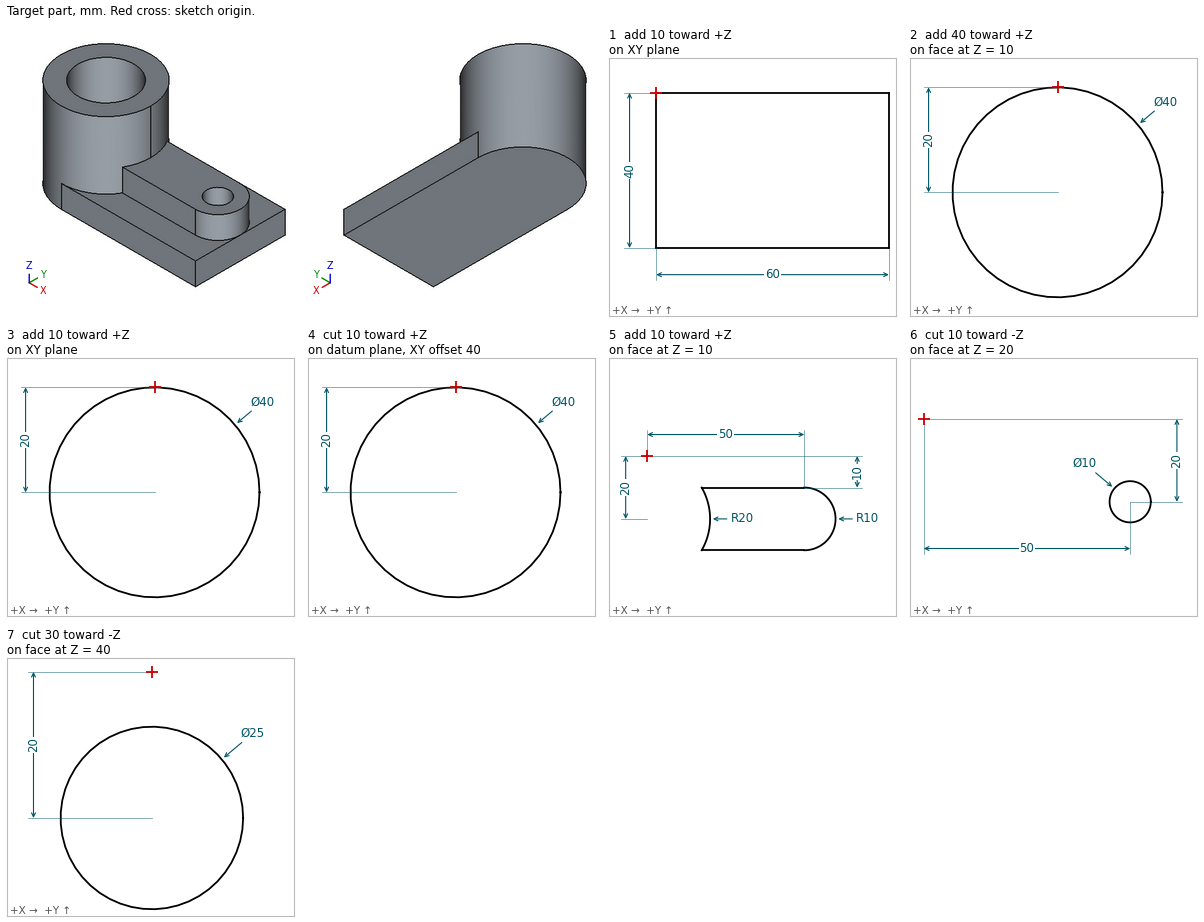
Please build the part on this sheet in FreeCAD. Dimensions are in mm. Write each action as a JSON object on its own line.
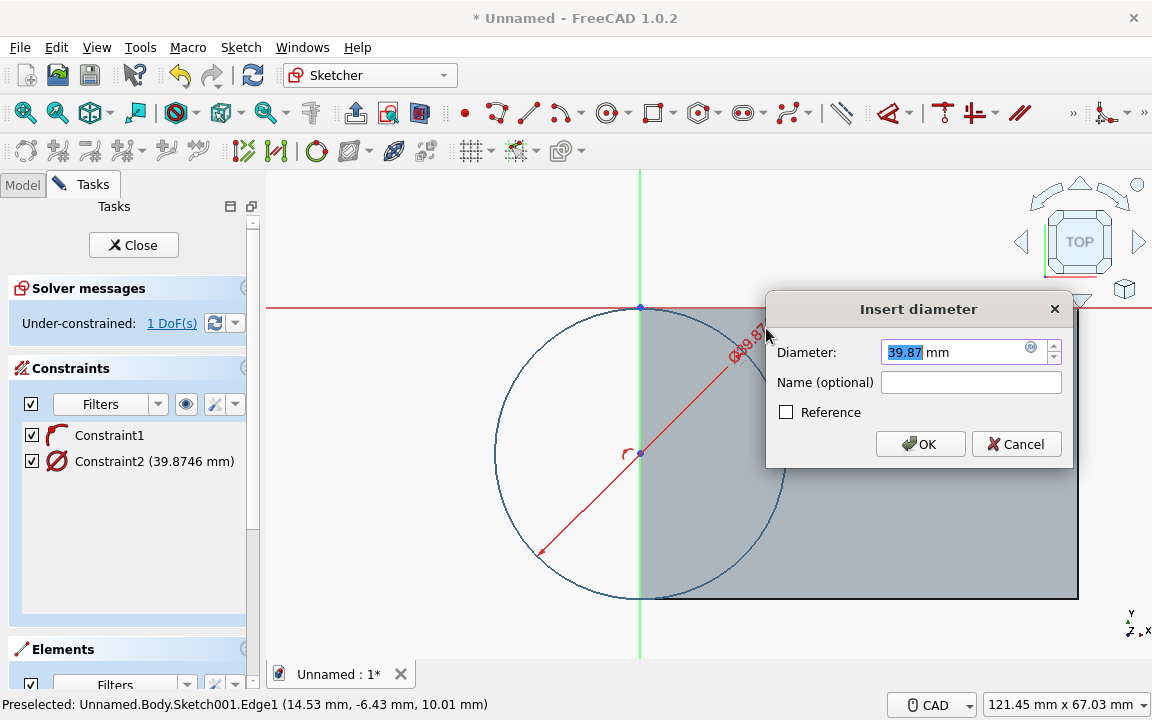
{"action": "type", "text": "40"}
{"action": "key", "text": "Return"}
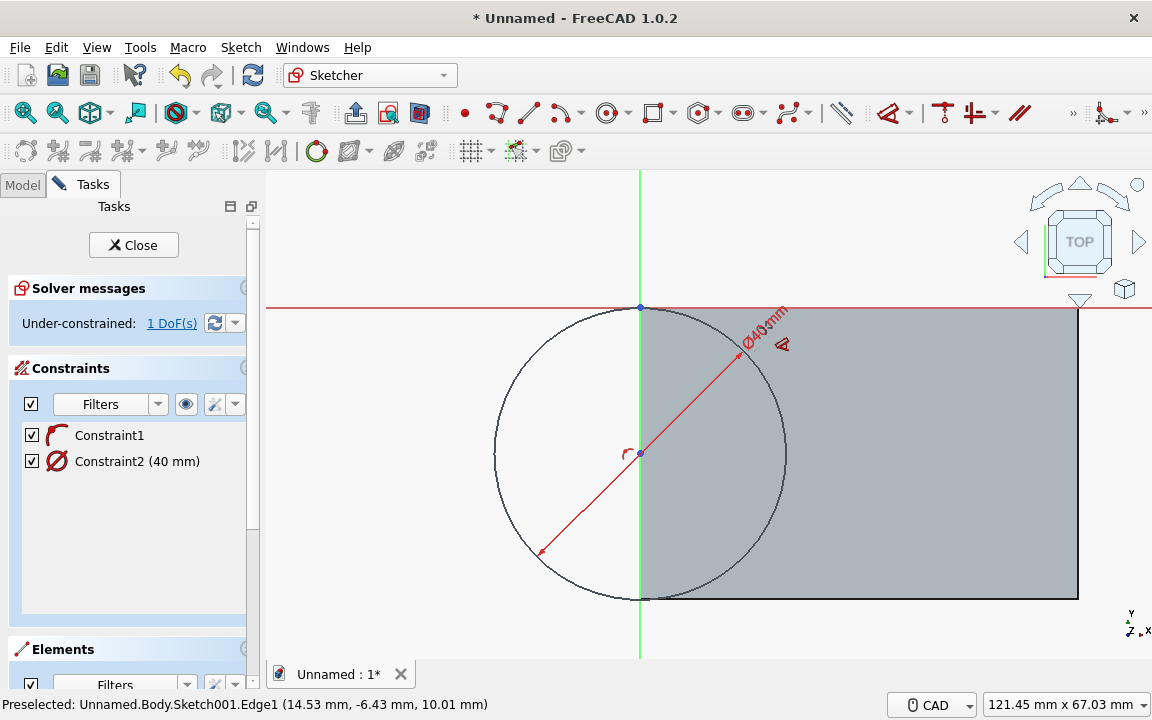
{"action": "left_click", "coordinate": [640, 454]}
{"action": "left_click", "coordinate": [674, 381]}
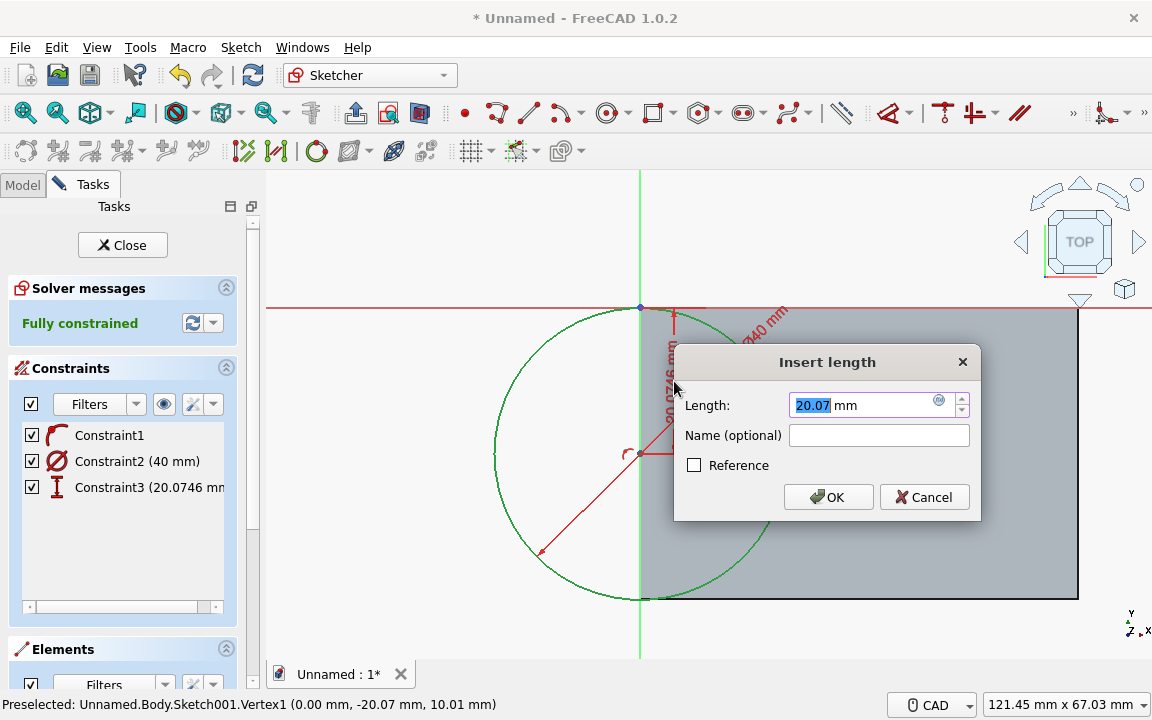
{"action": "type", "text": "20"}
{"action": "key", "text": "Return"}
{"action": "key", "text": "Escape"}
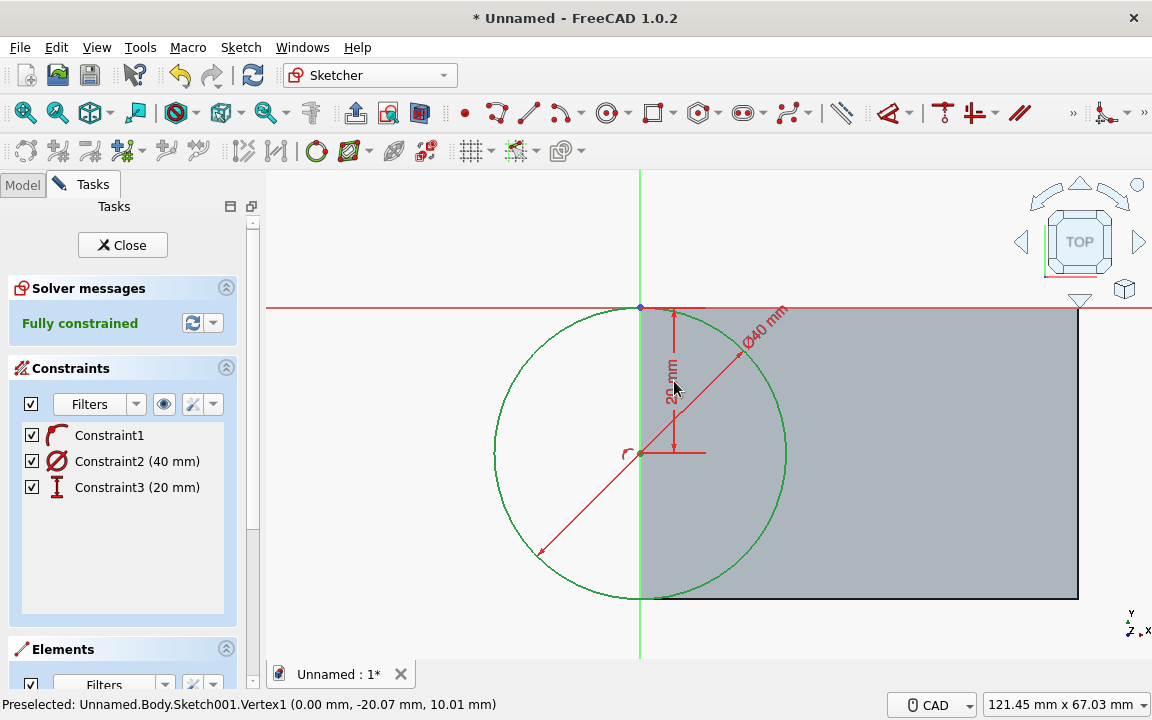
{"action": "left_click", "coordinate": [123, 245]}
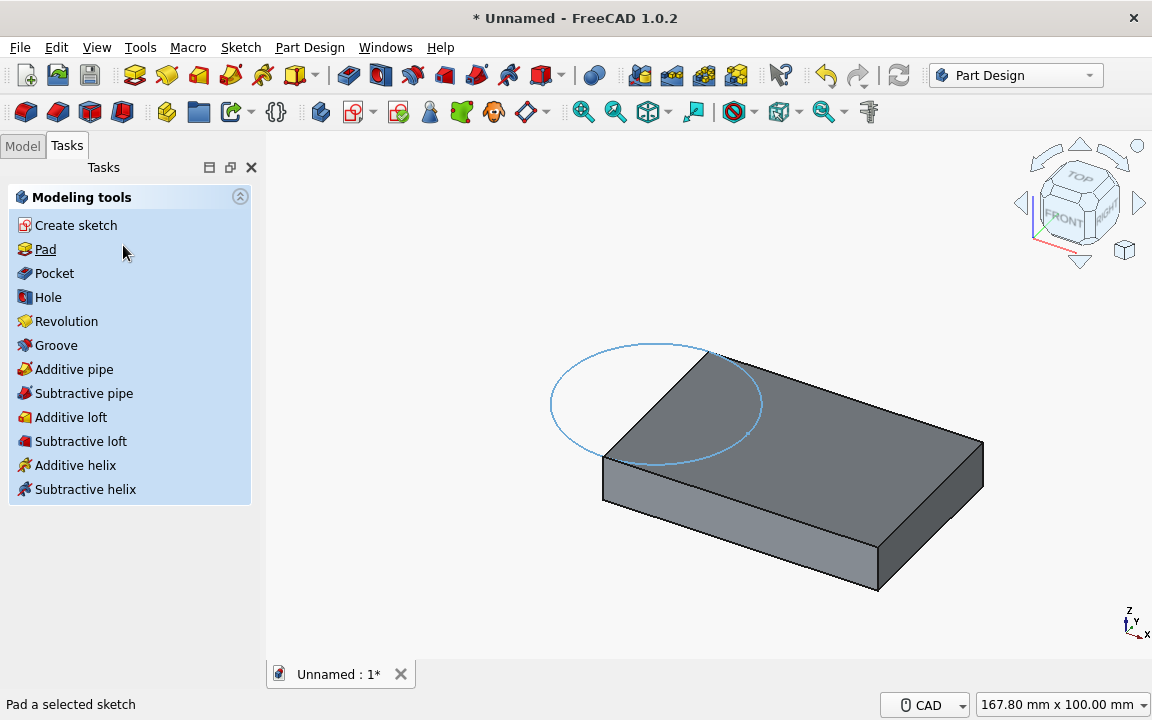
{"action": "left_click", "coordinate": [136, 76]}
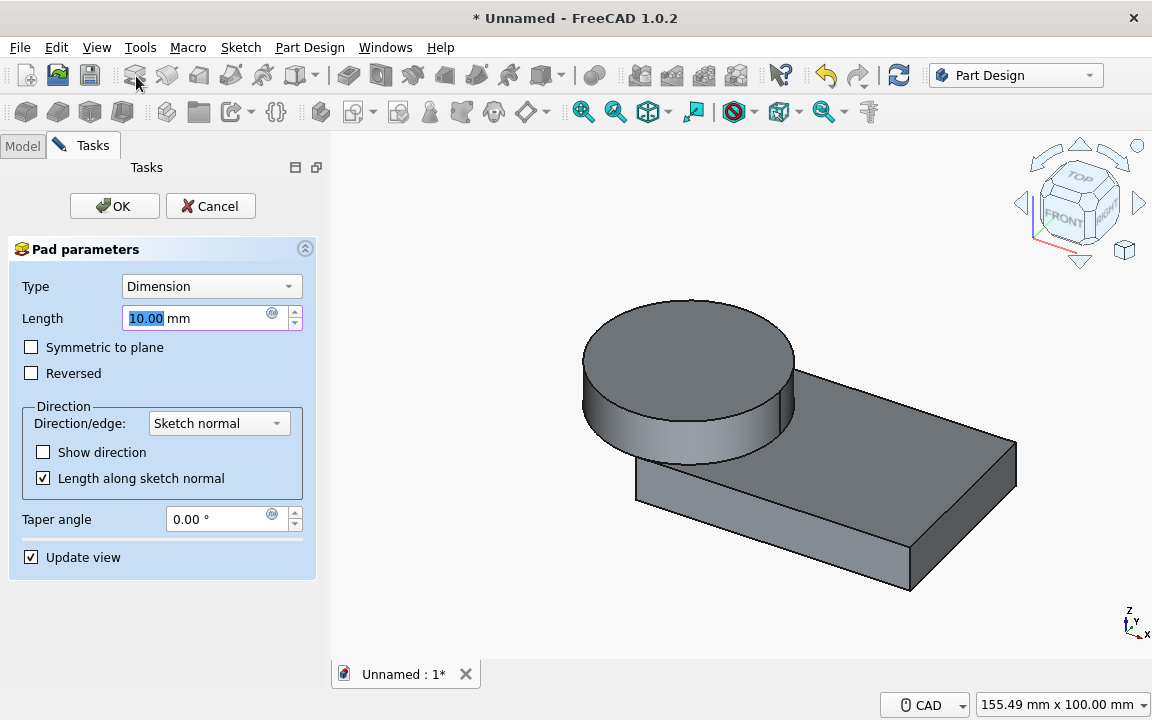
{"action": "type", "text": "40"}
{"action": "key", "text": "Tab"}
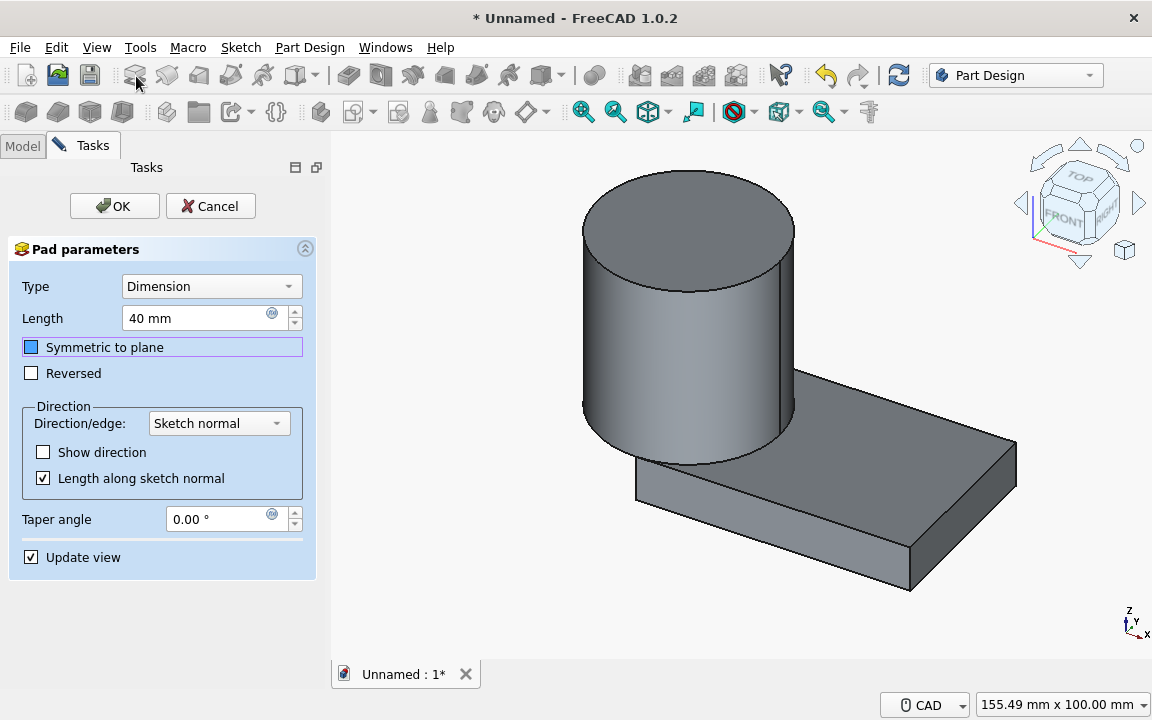
{"action": "left_click", "coordinate": [115, 206]}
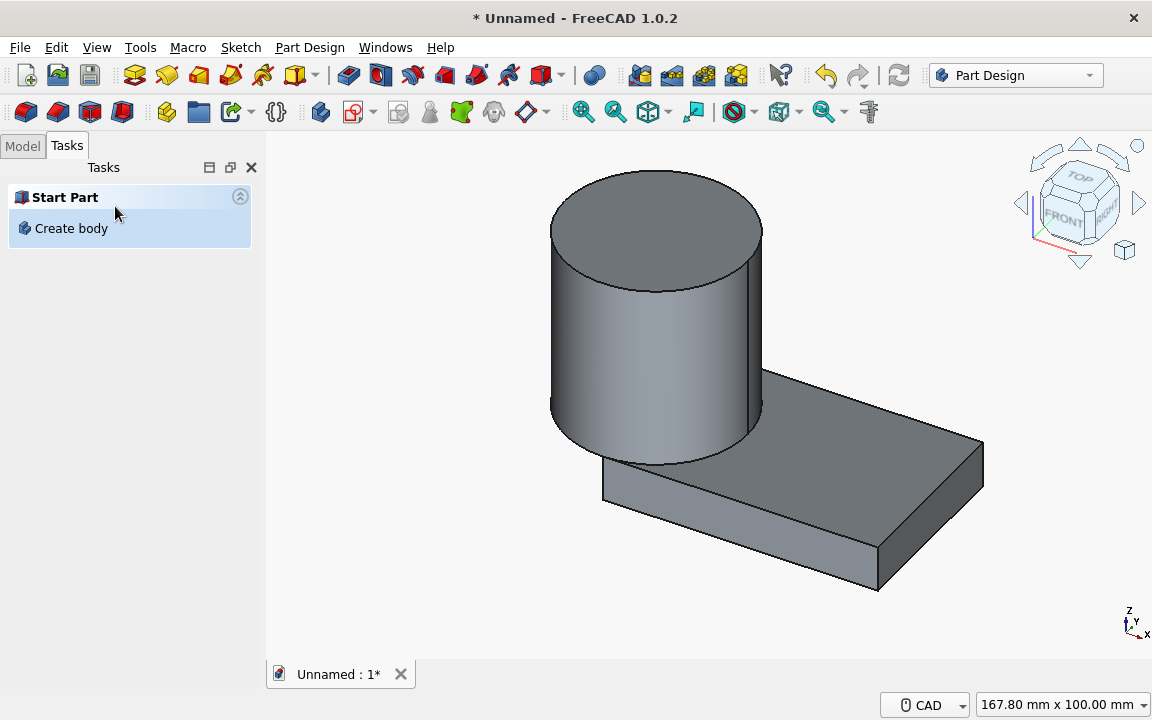
{"action": "left_click", "coordinate": [354, 112]}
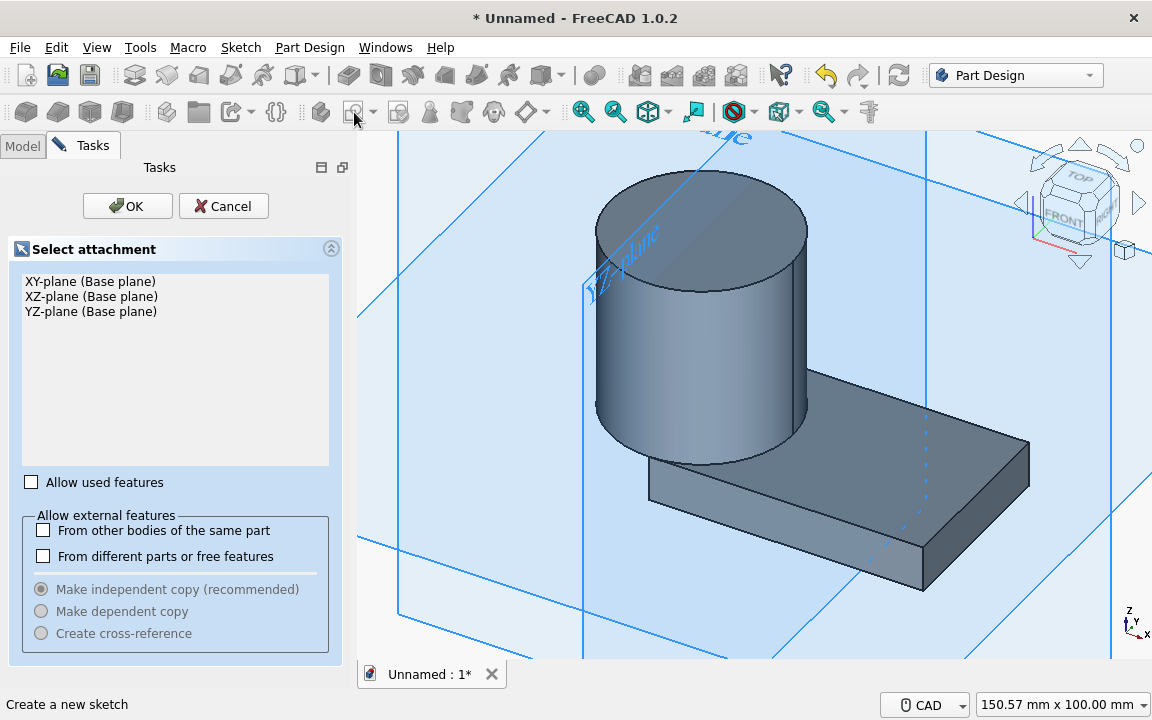
{"action": "left_click", "coordinate": [82, 282]}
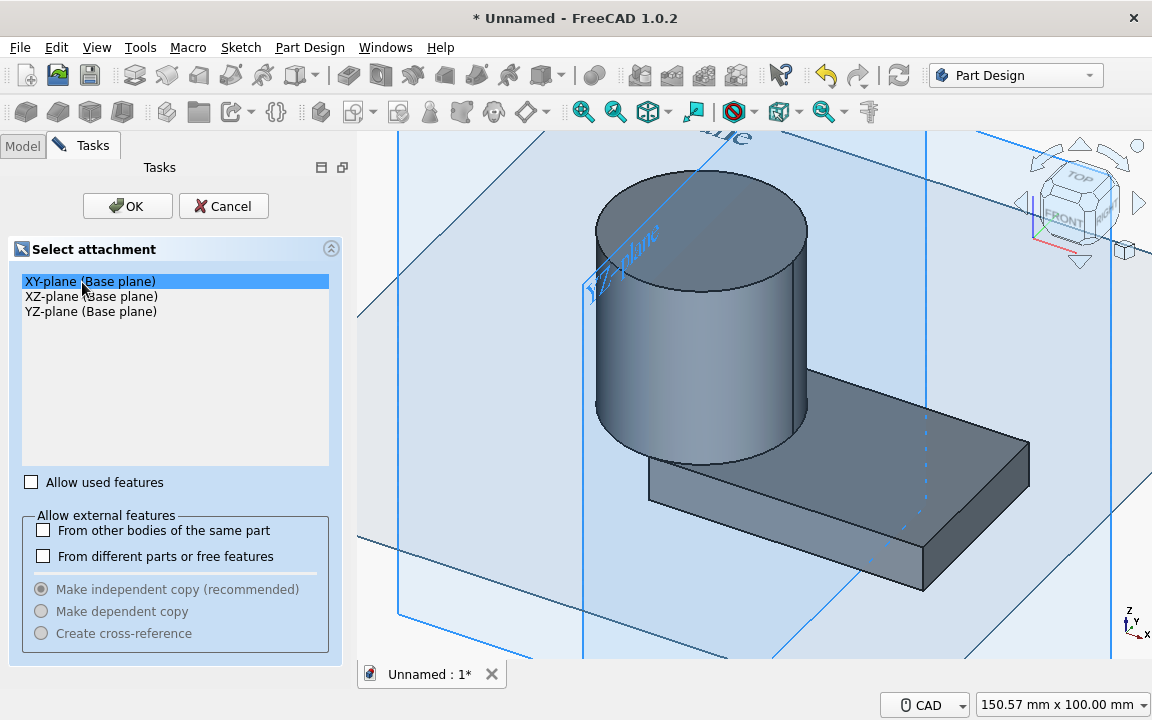
{"action": "left_click", "coordinate": [128, 206]}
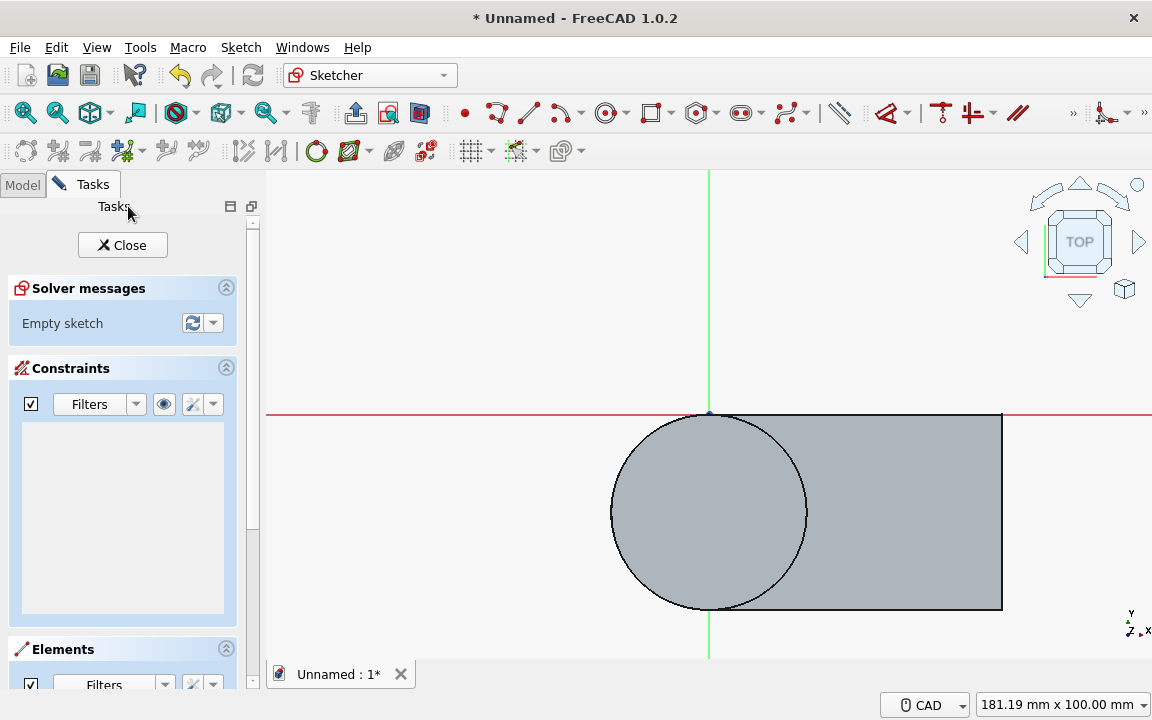
{"action": "left_click", "coordinate": [420, 114]}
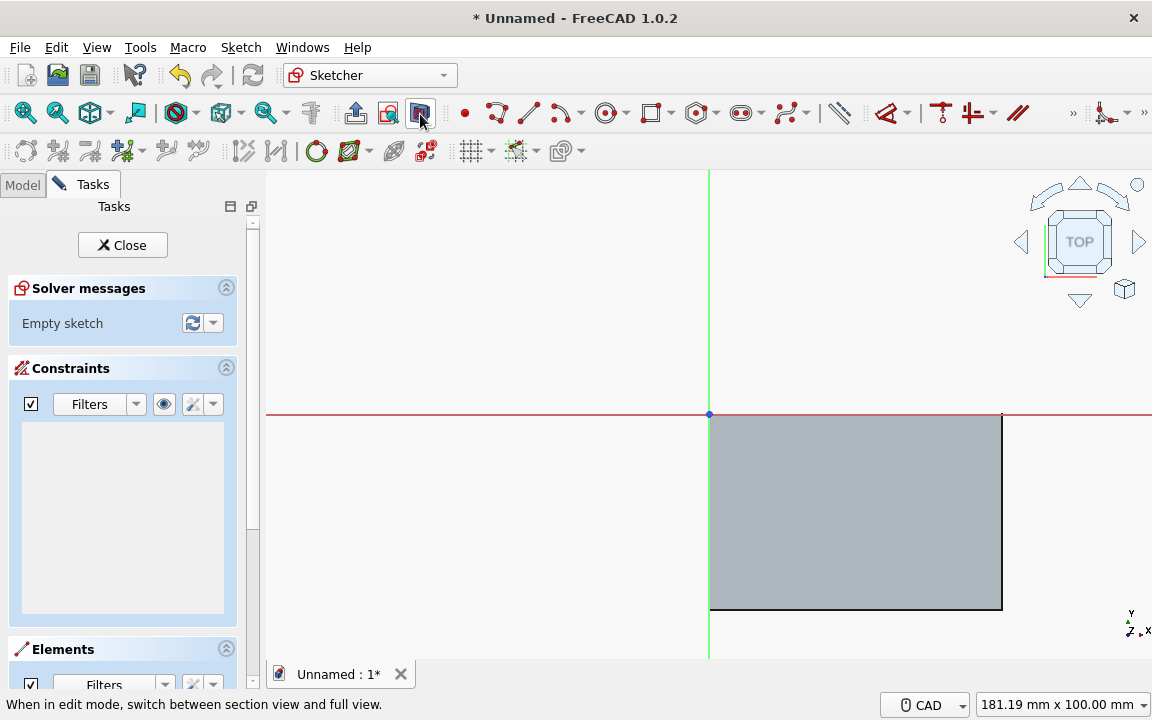
{"action": "scroll", "coordinate": [848, 631], "scroll_direction": "up", "scroll_amount": 2}